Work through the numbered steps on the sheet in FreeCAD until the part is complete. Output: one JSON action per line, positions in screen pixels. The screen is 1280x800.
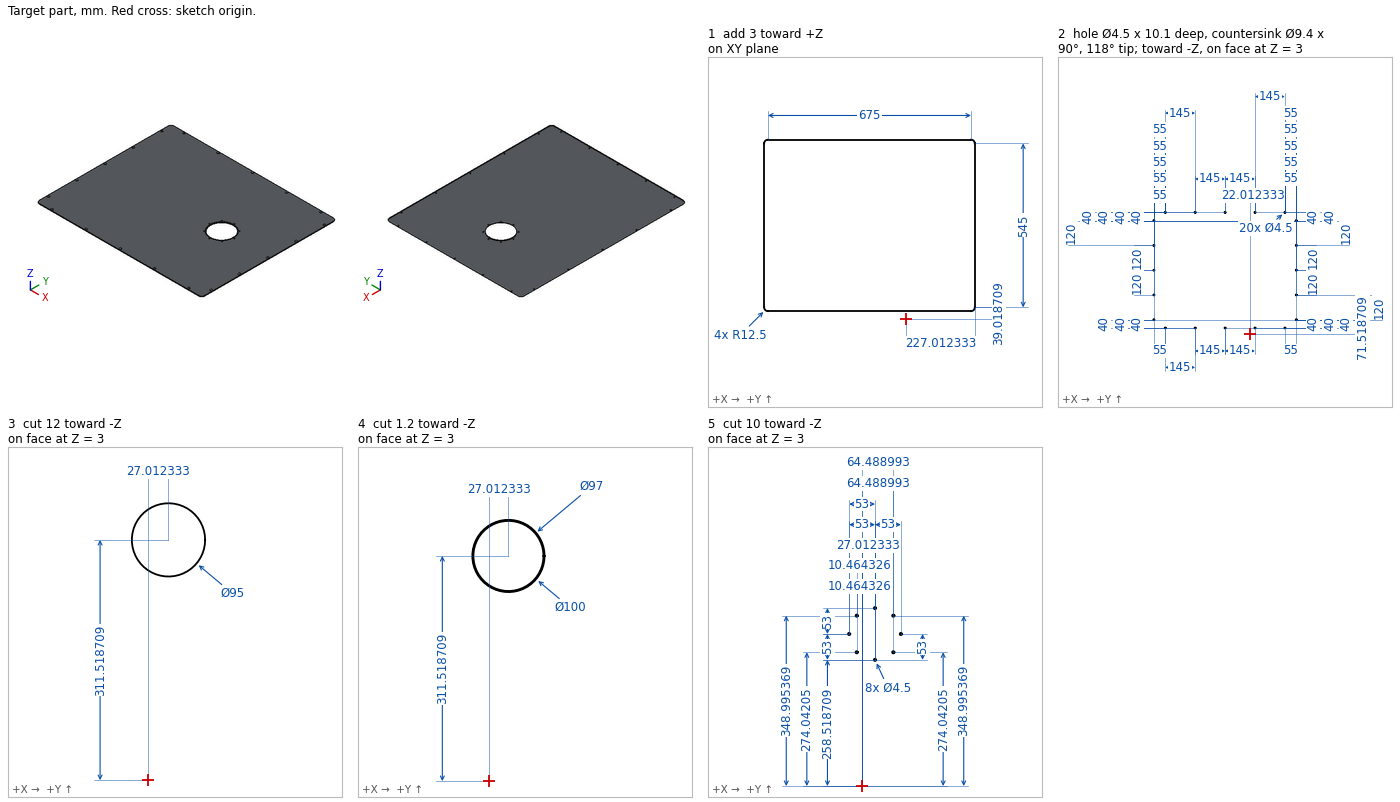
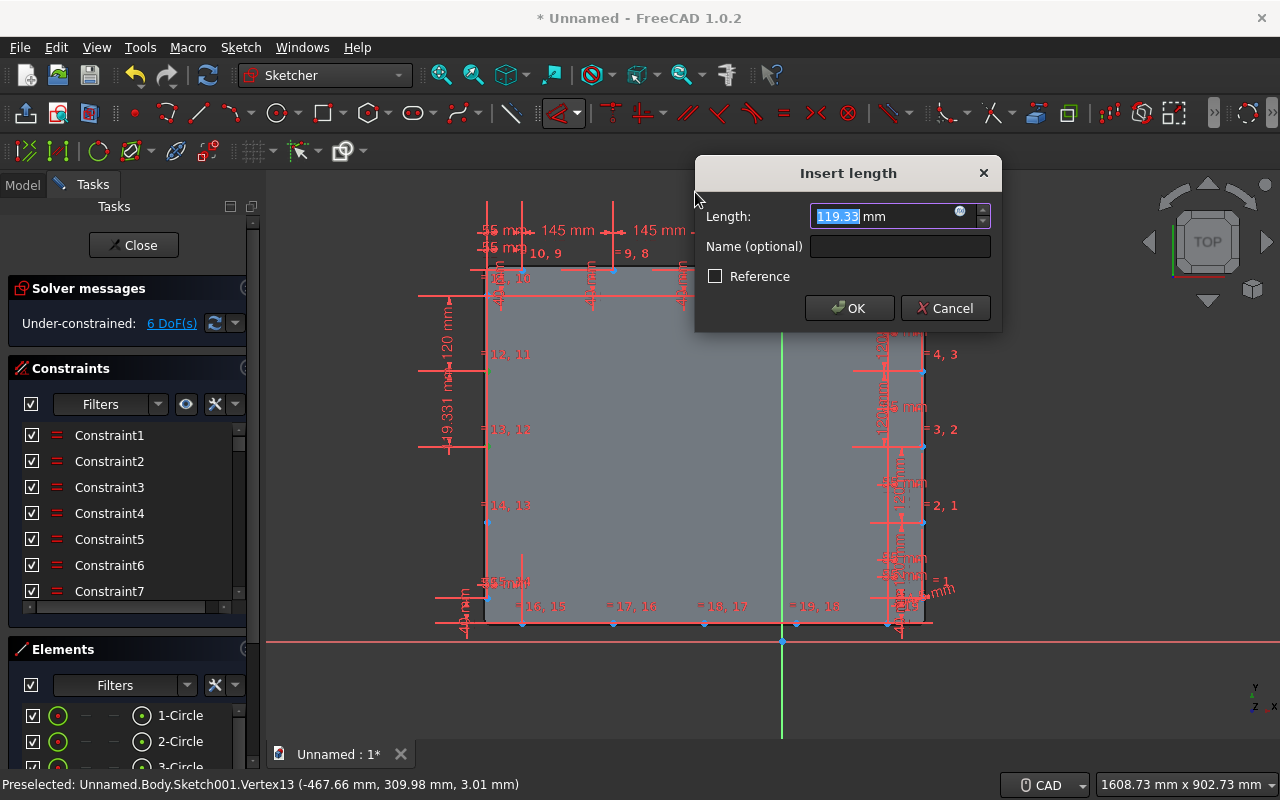
{"action": "type", "text": "120"}
{"action": "key", "text": "Return"}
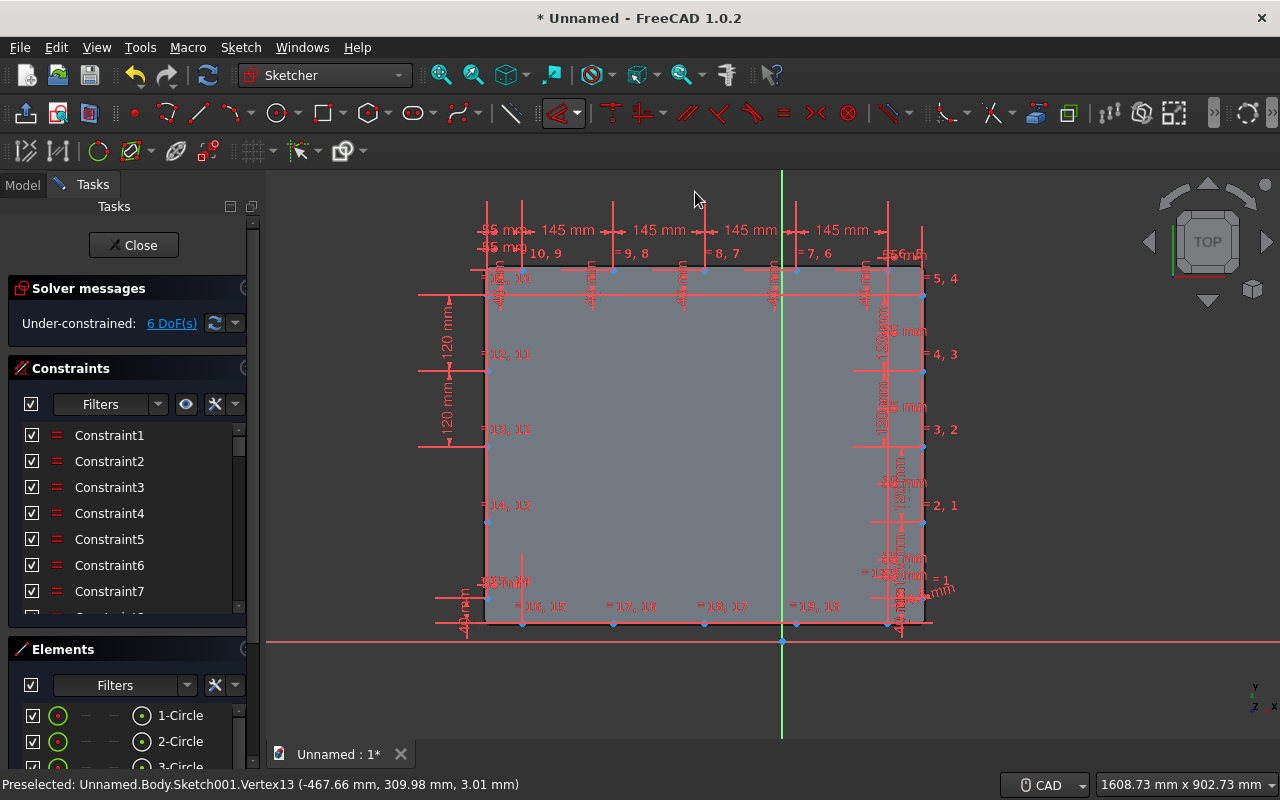
{"action": "left_click", "coordinate": [487, 447]}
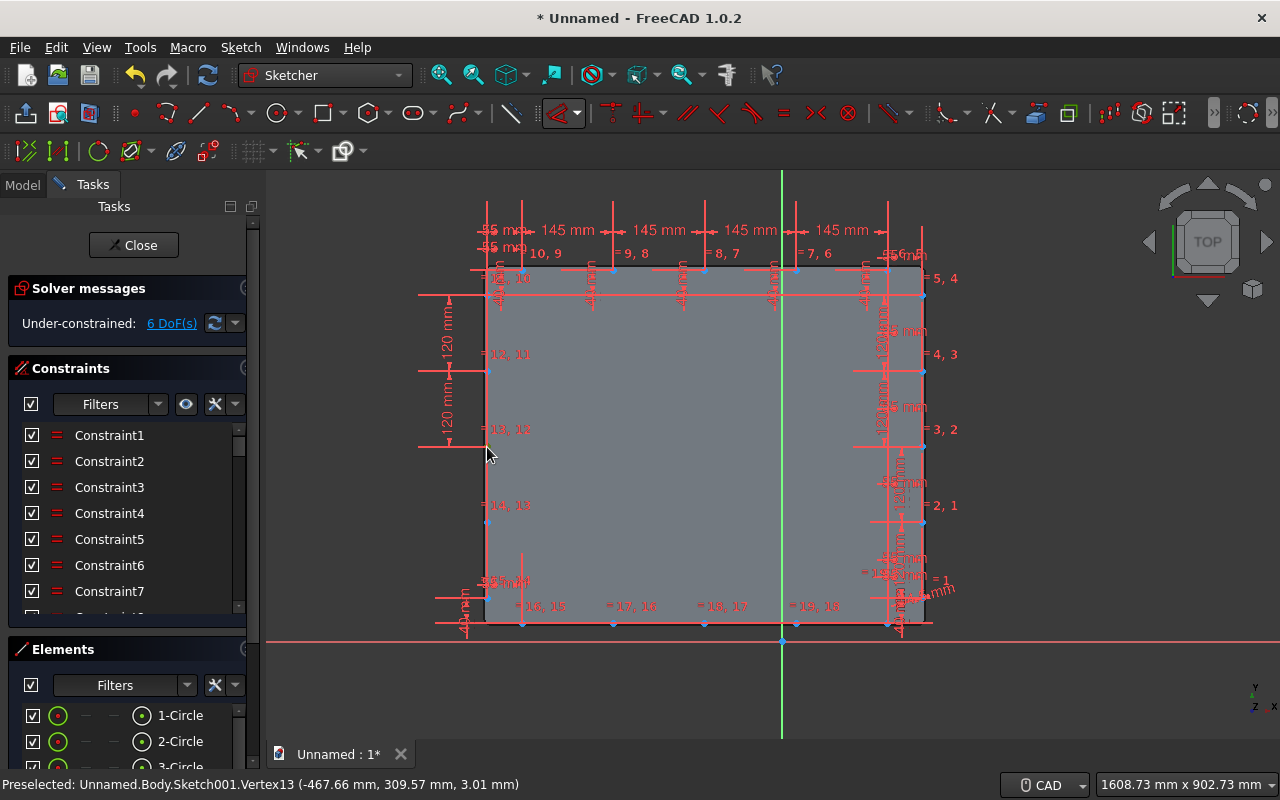
{"action": "left_click", "coordinate": [487, 522]}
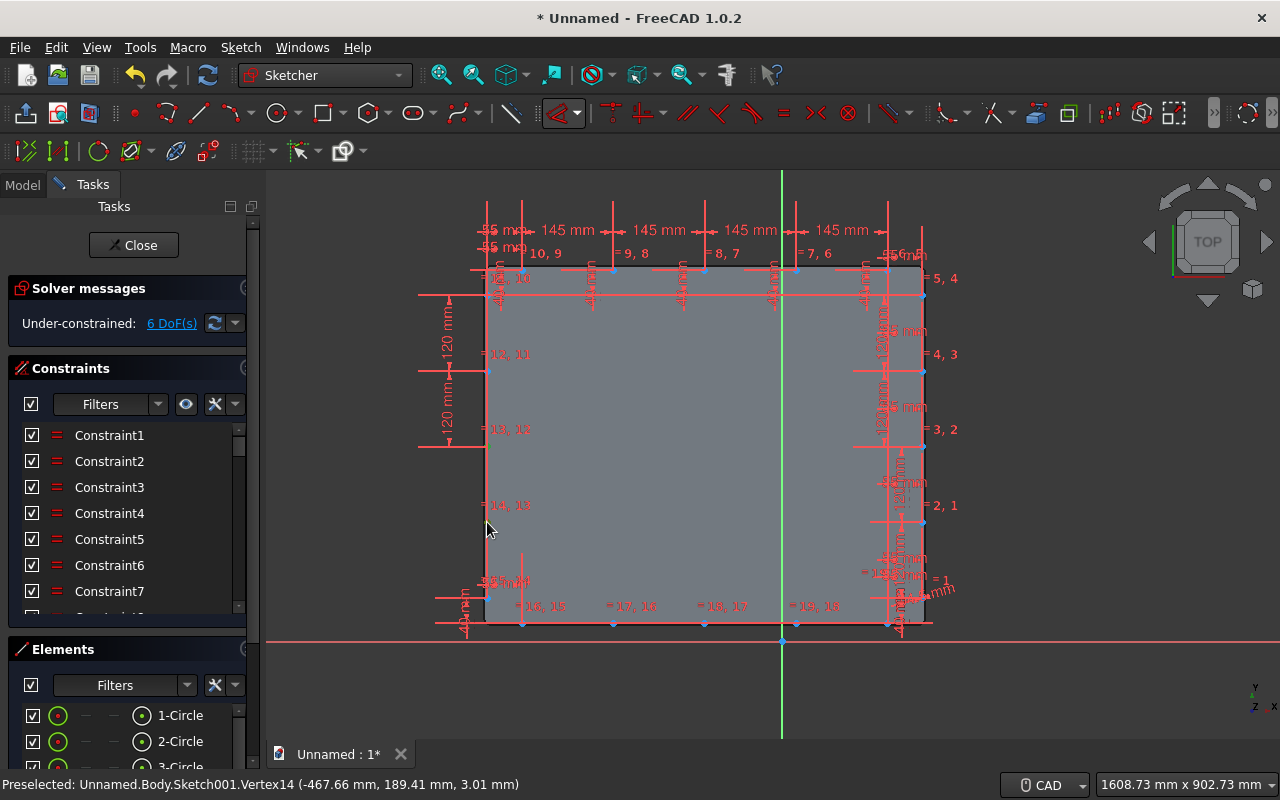
{"action": "left_click", "coordinate": [580, 114]}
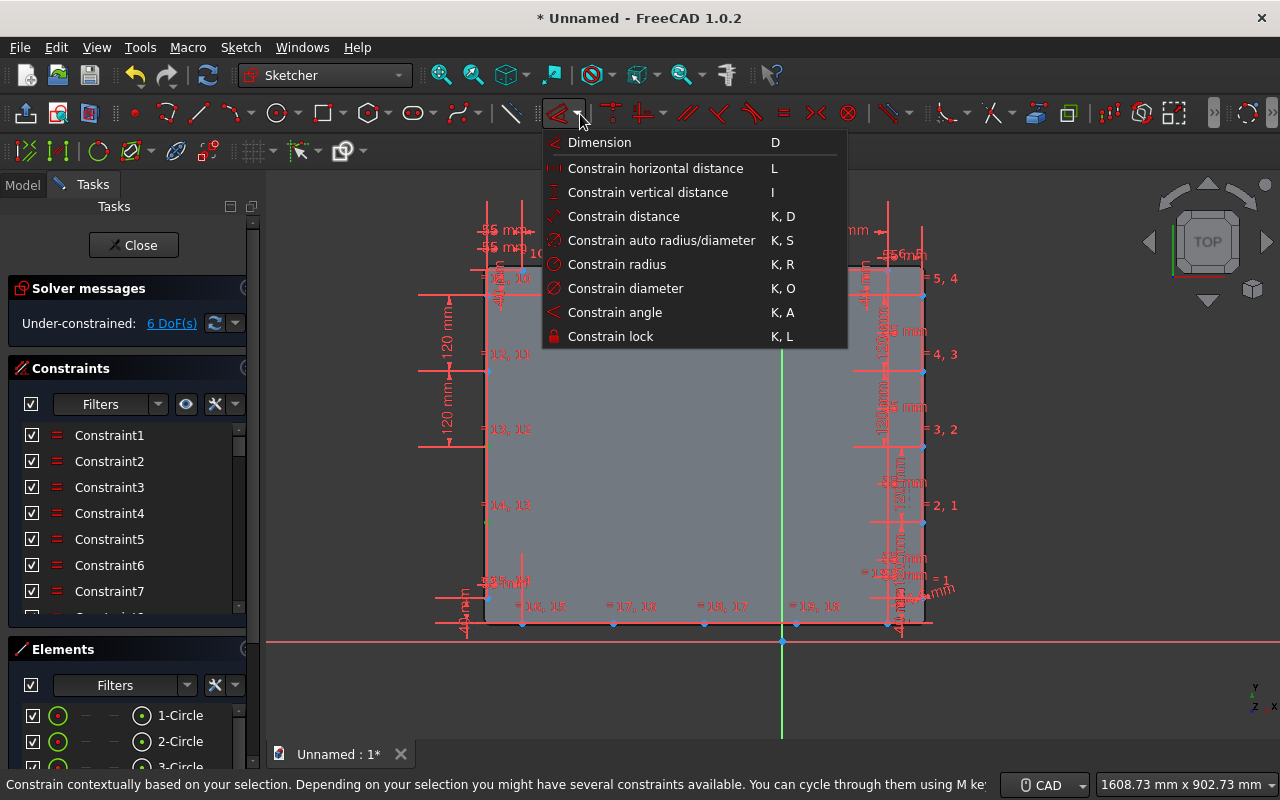
{"action": "left_click", "coordinate": [695, 192]}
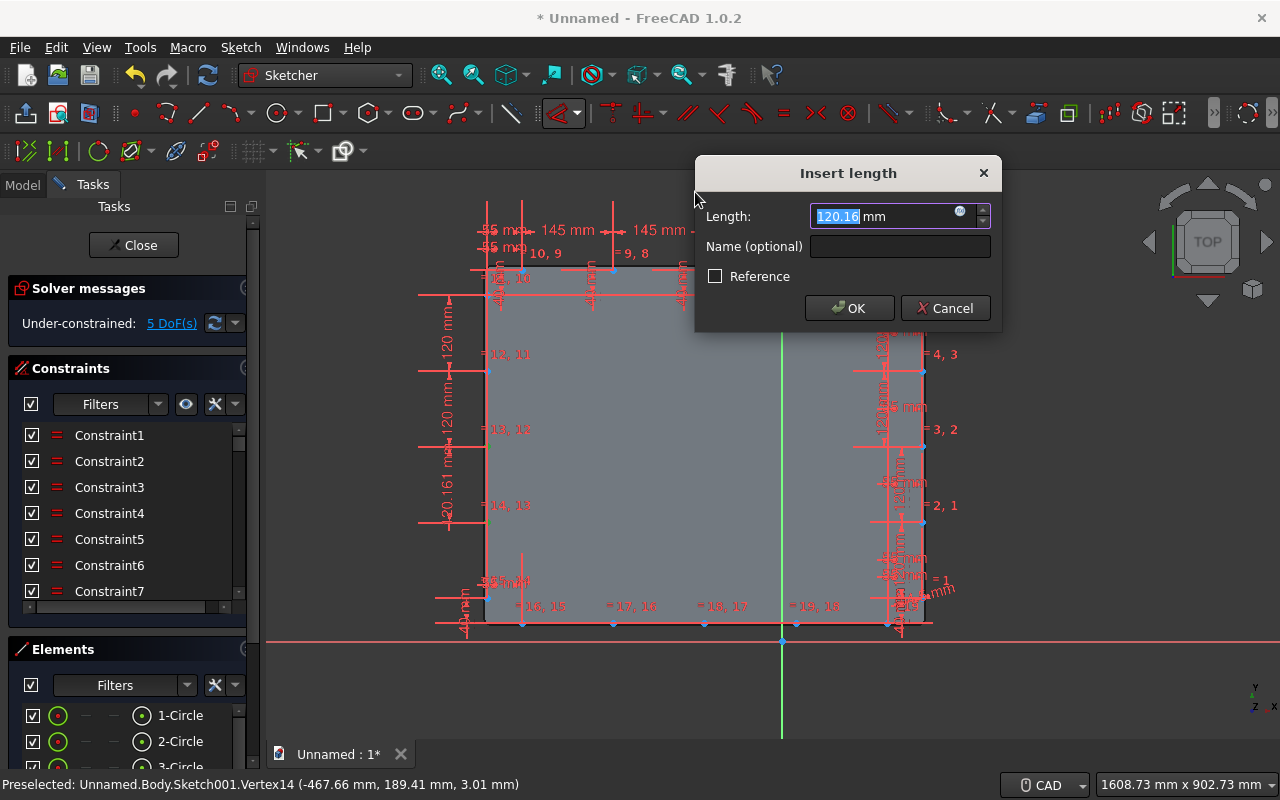
{"action": "type", "text": "120"}
{"action": "key", "text": "Return"}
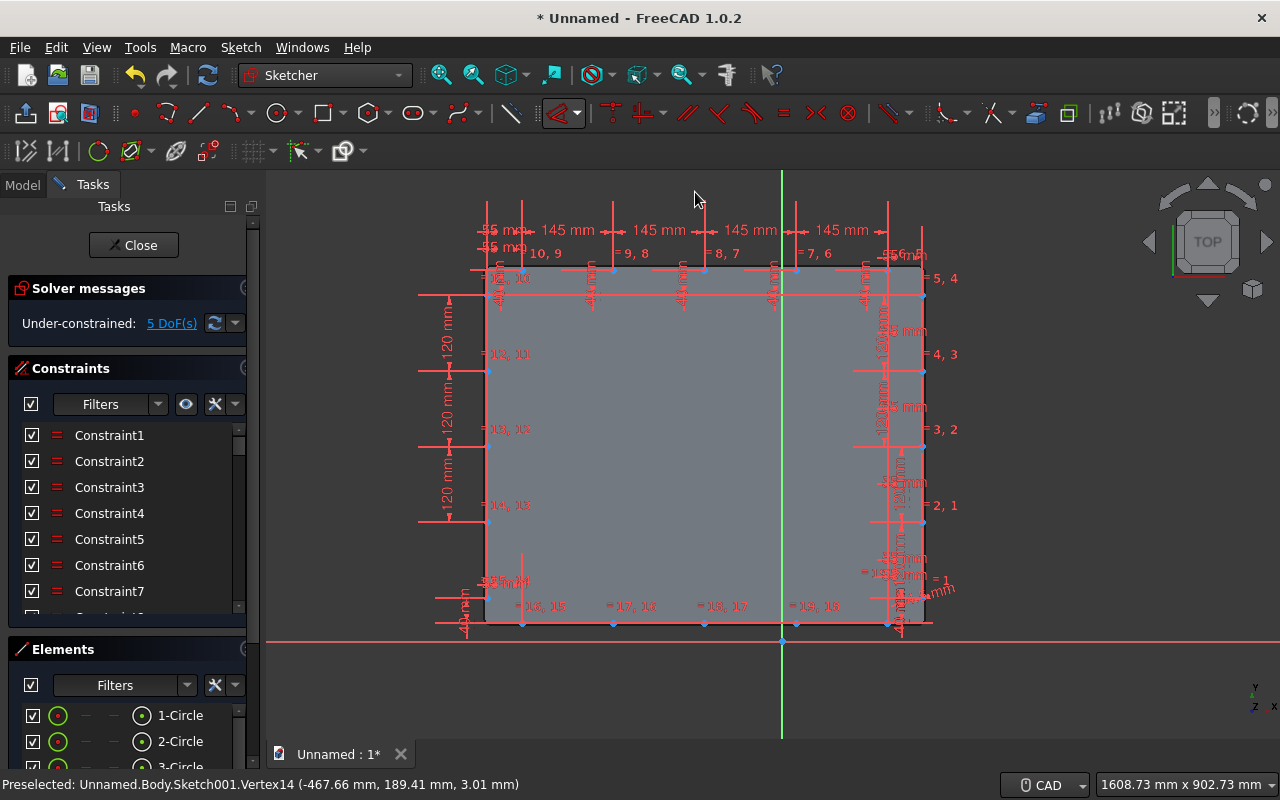
{"action": "left_click", "coordinate": [522, 623]}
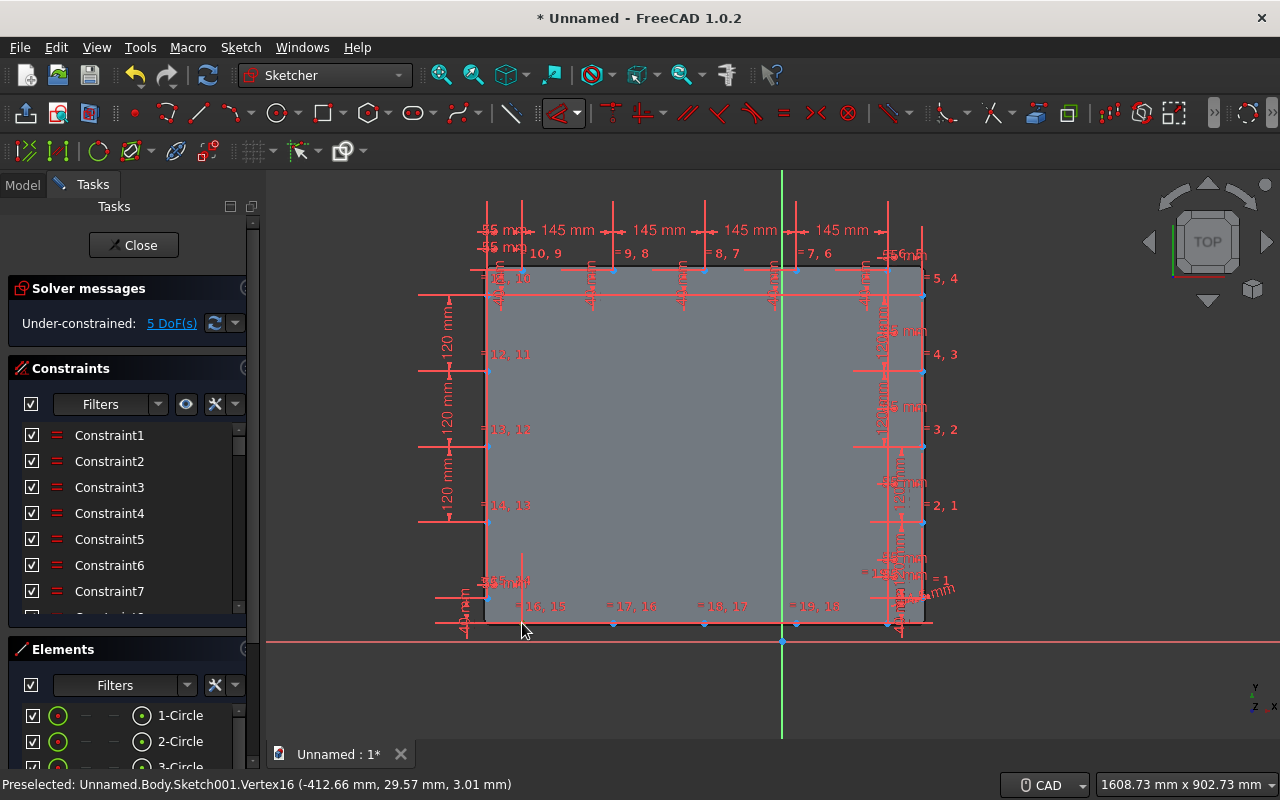
{"action": "left_click", "coordinate": [613, 623]}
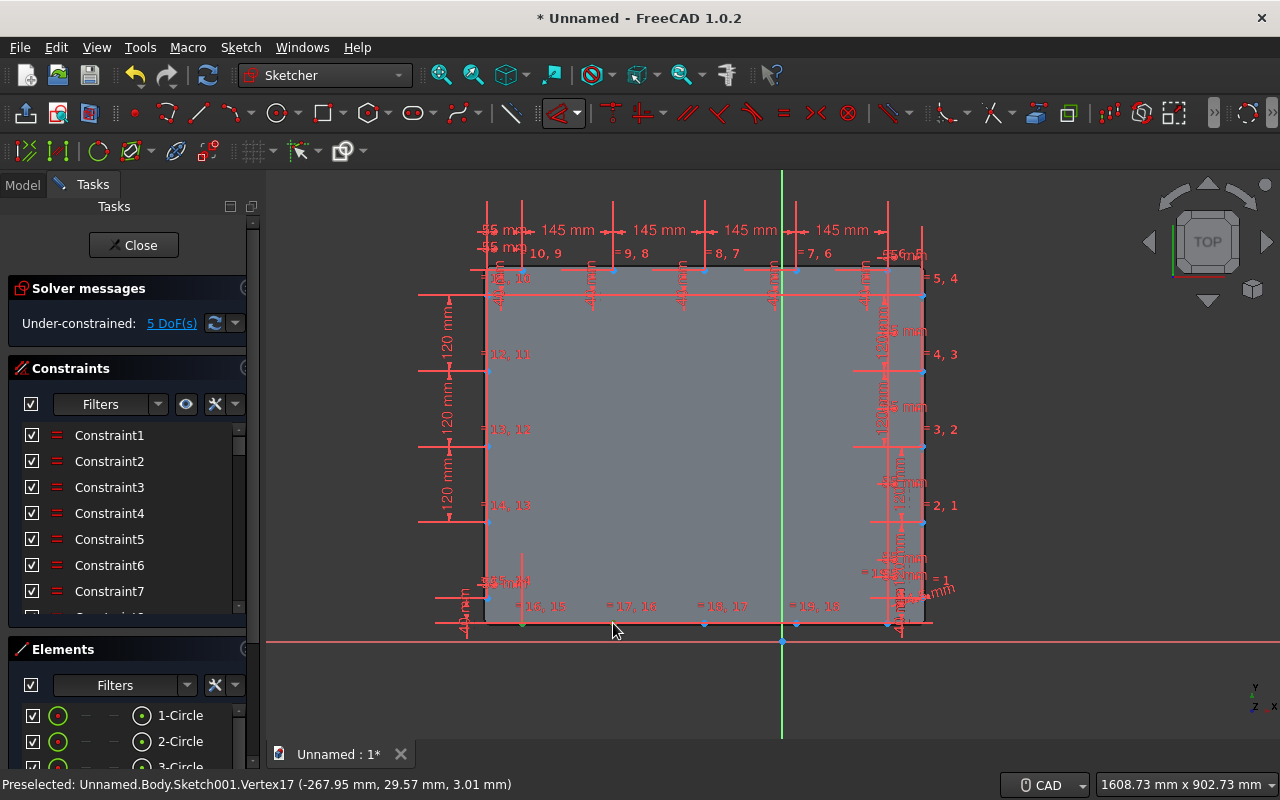
{"action": "left_click", "coordinate": [580, 114]}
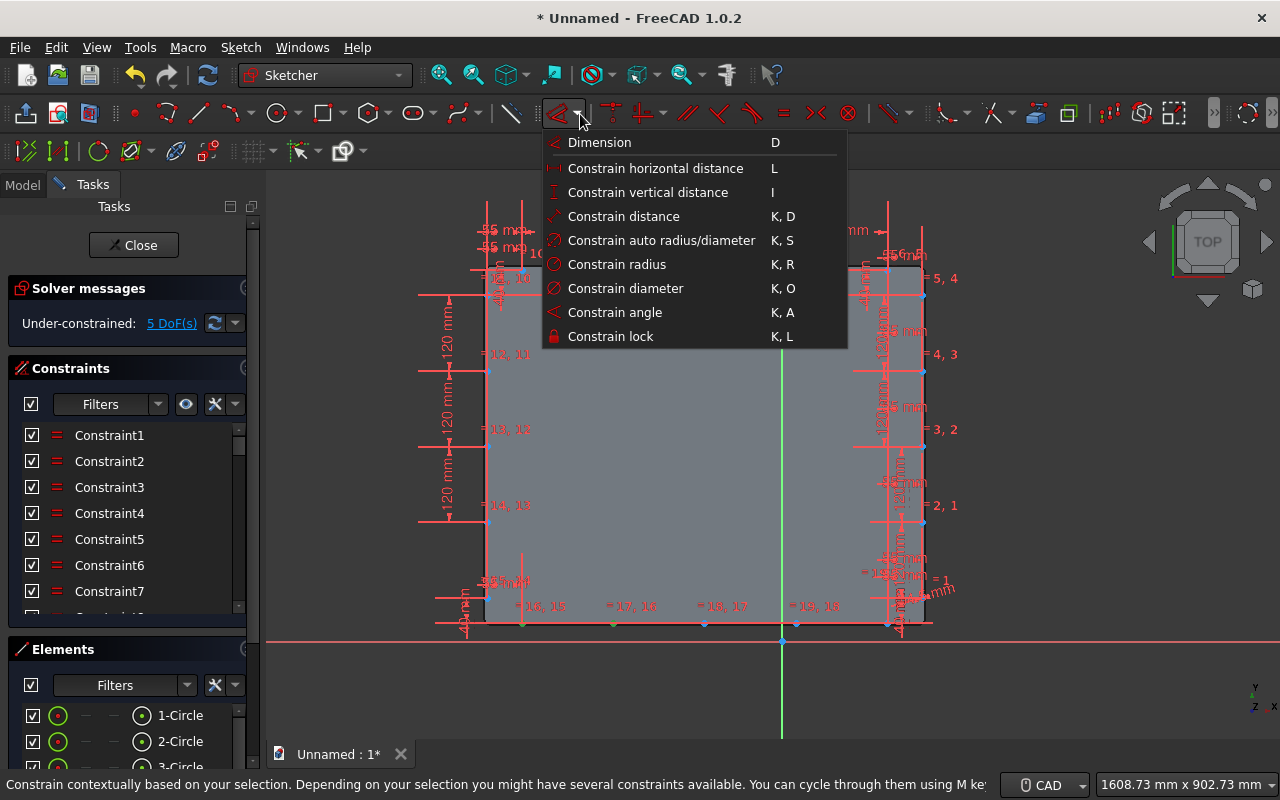
{"action": "left_click", "coordinate": [695, 168]}